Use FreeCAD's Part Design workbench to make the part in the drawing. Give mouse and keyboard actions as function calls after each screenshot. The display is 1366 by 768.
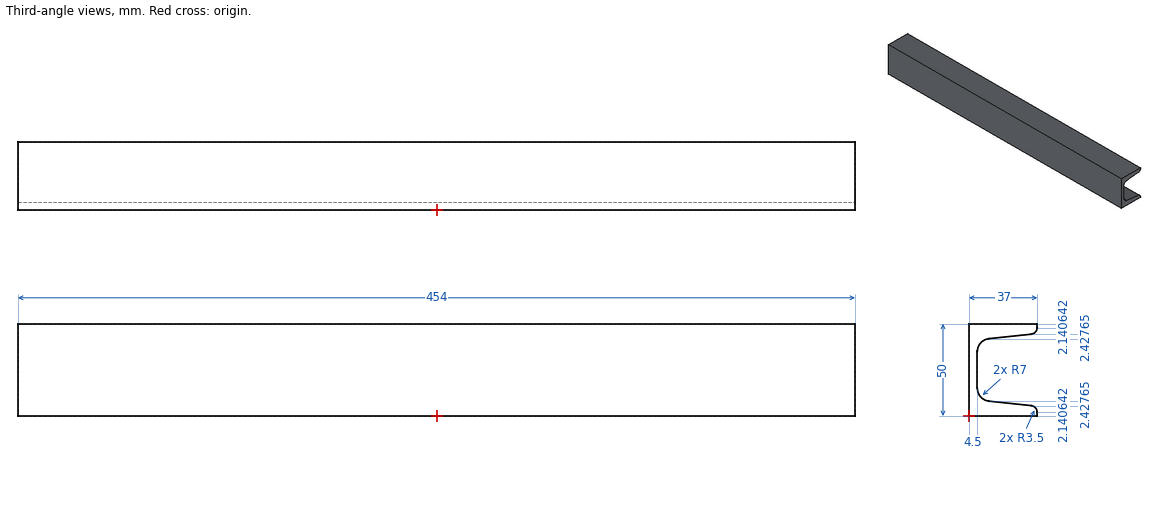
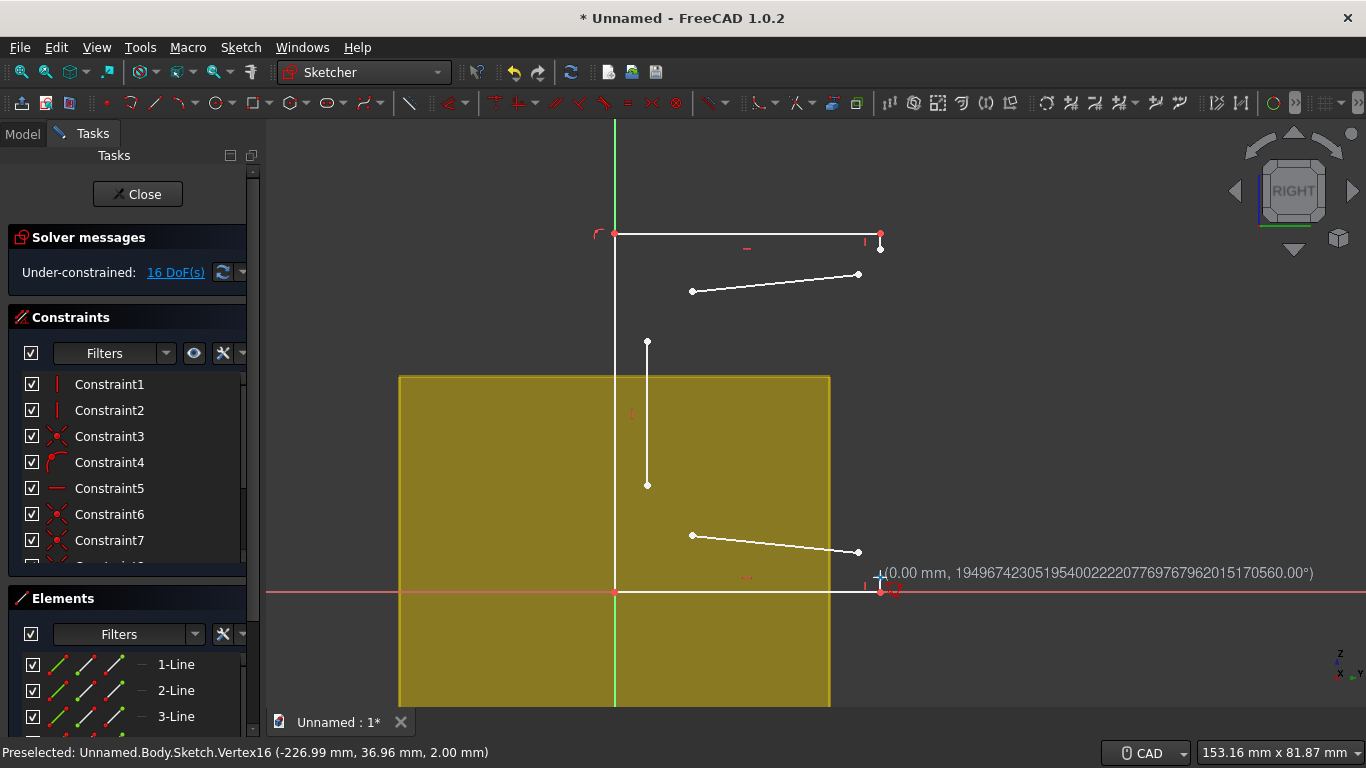
click(180, 104)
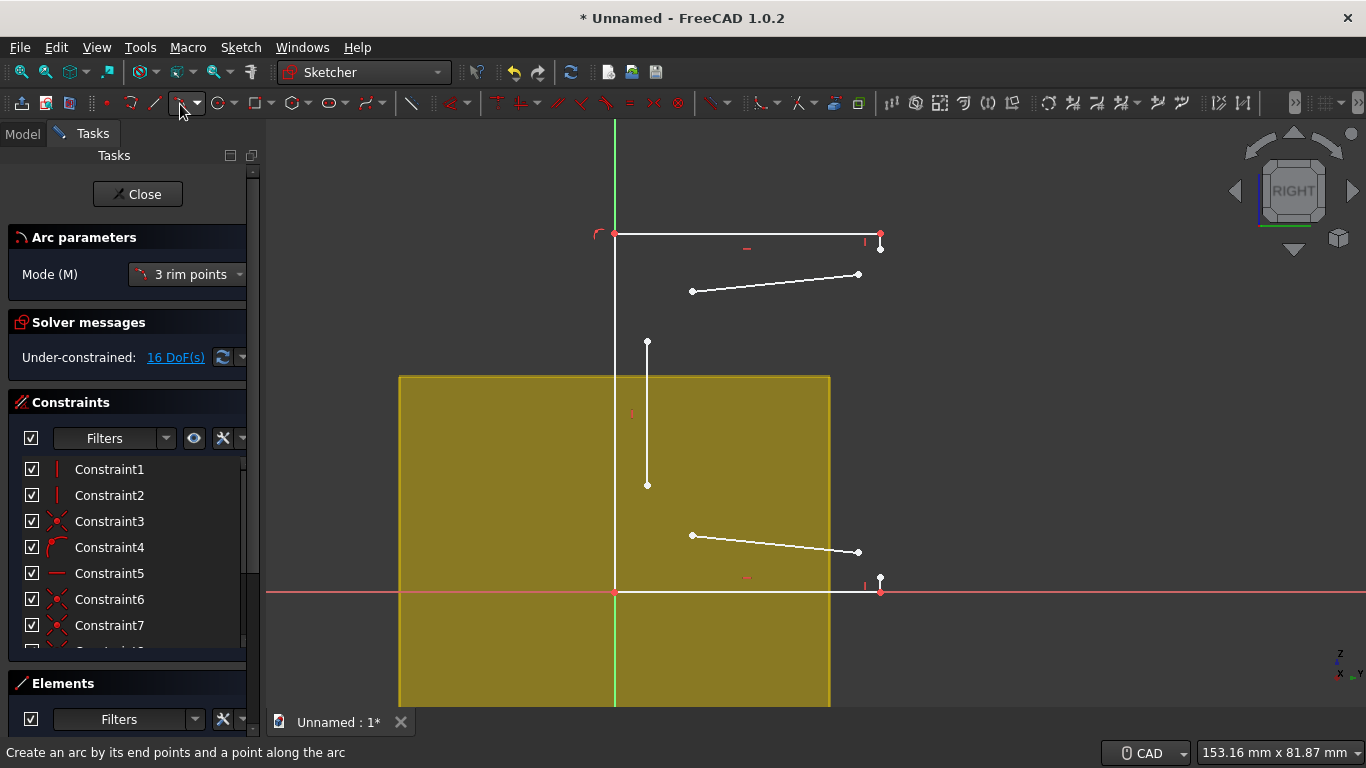
click(692, 536)
click(647, 486)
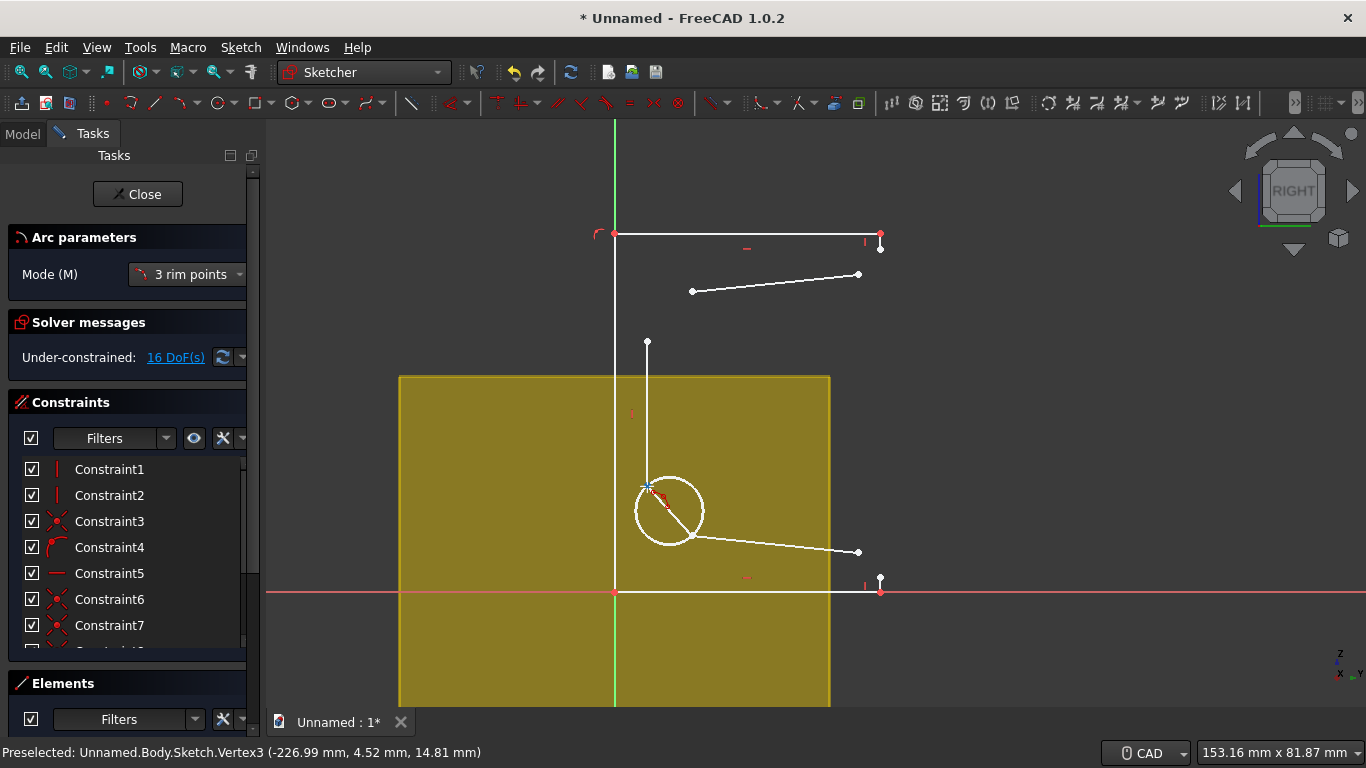
scroll(660, 518, up, 2)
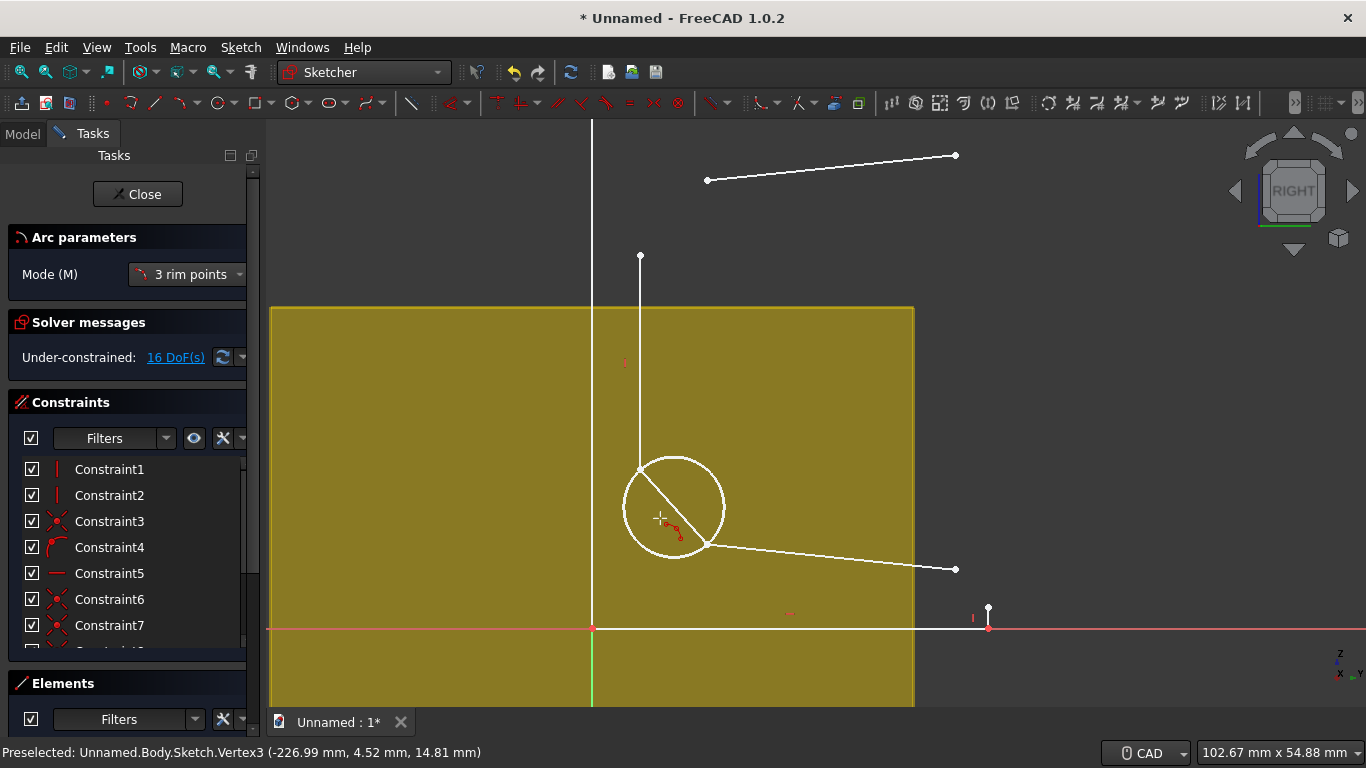
click(659, 518)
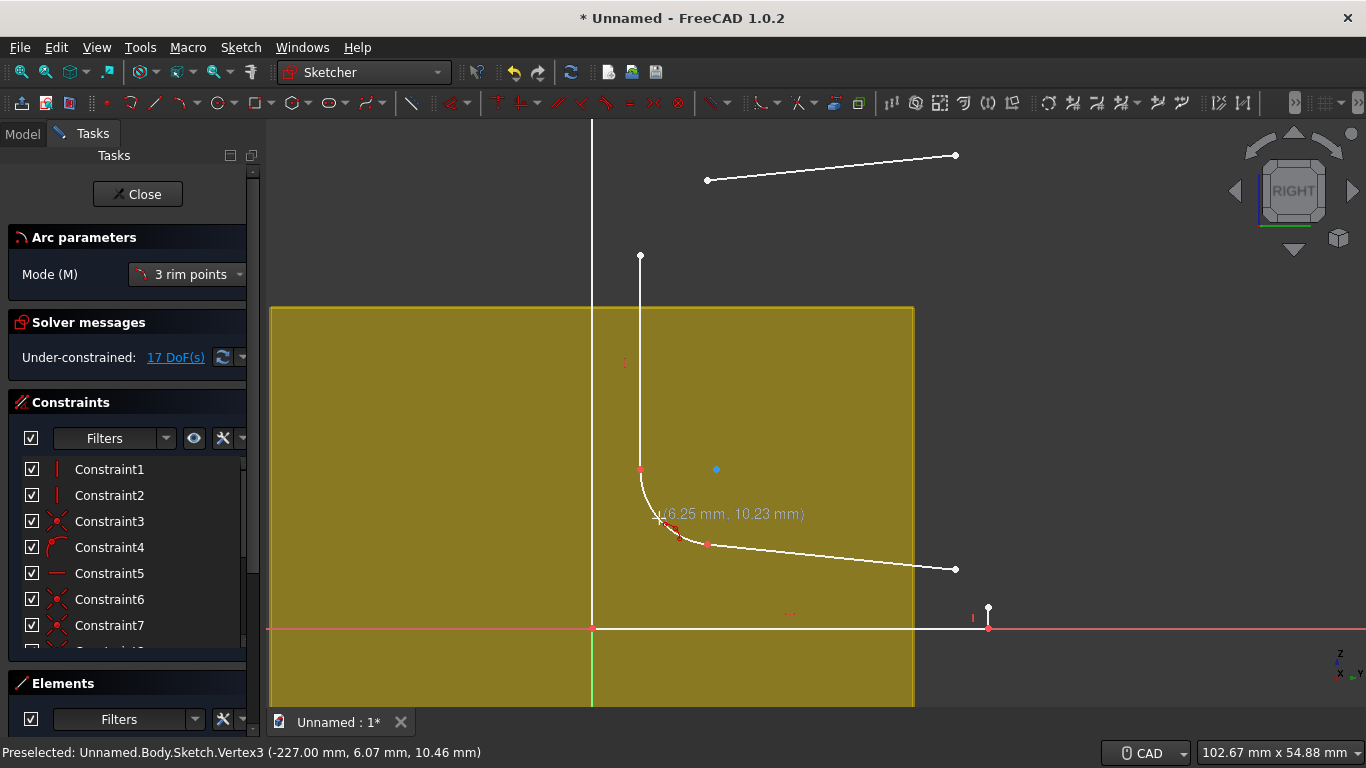
click(640, 255)
click(708, 181)
click(659, 204)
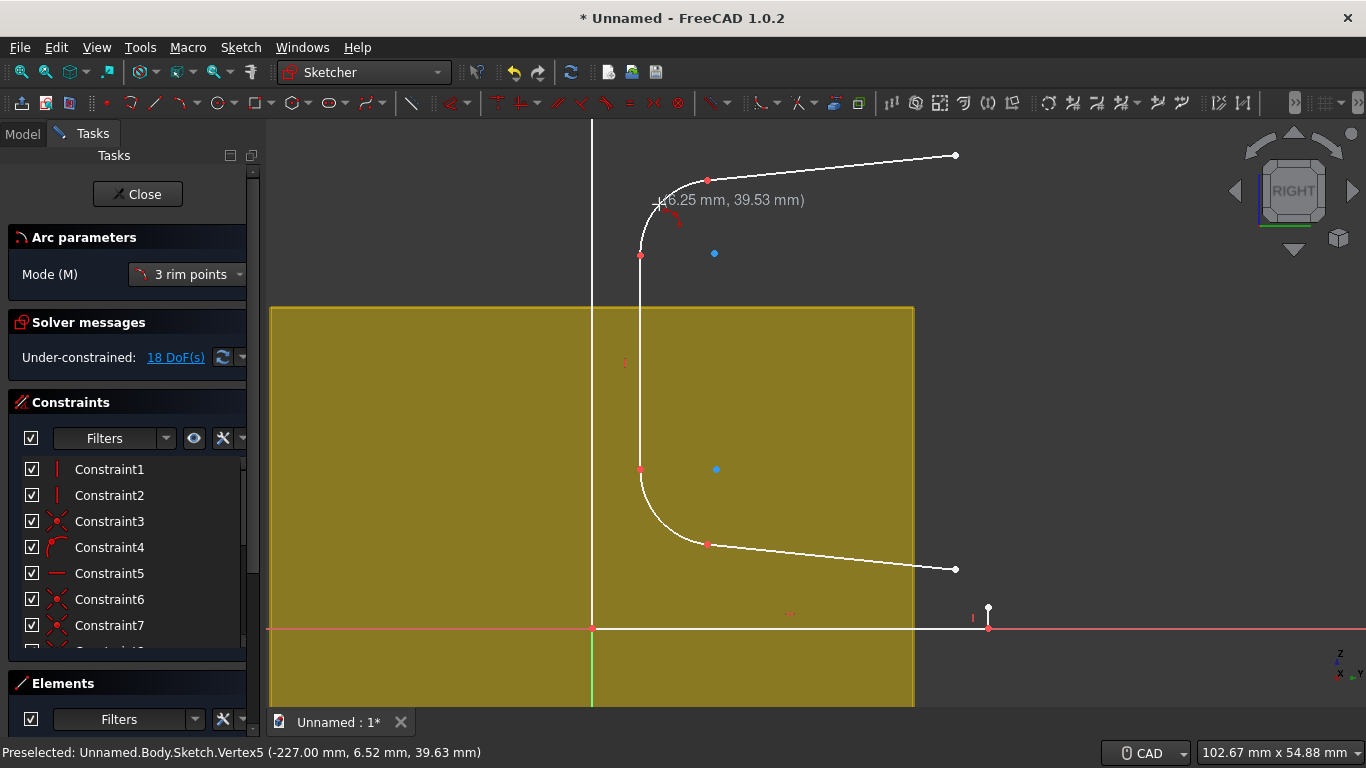
click(955, 155)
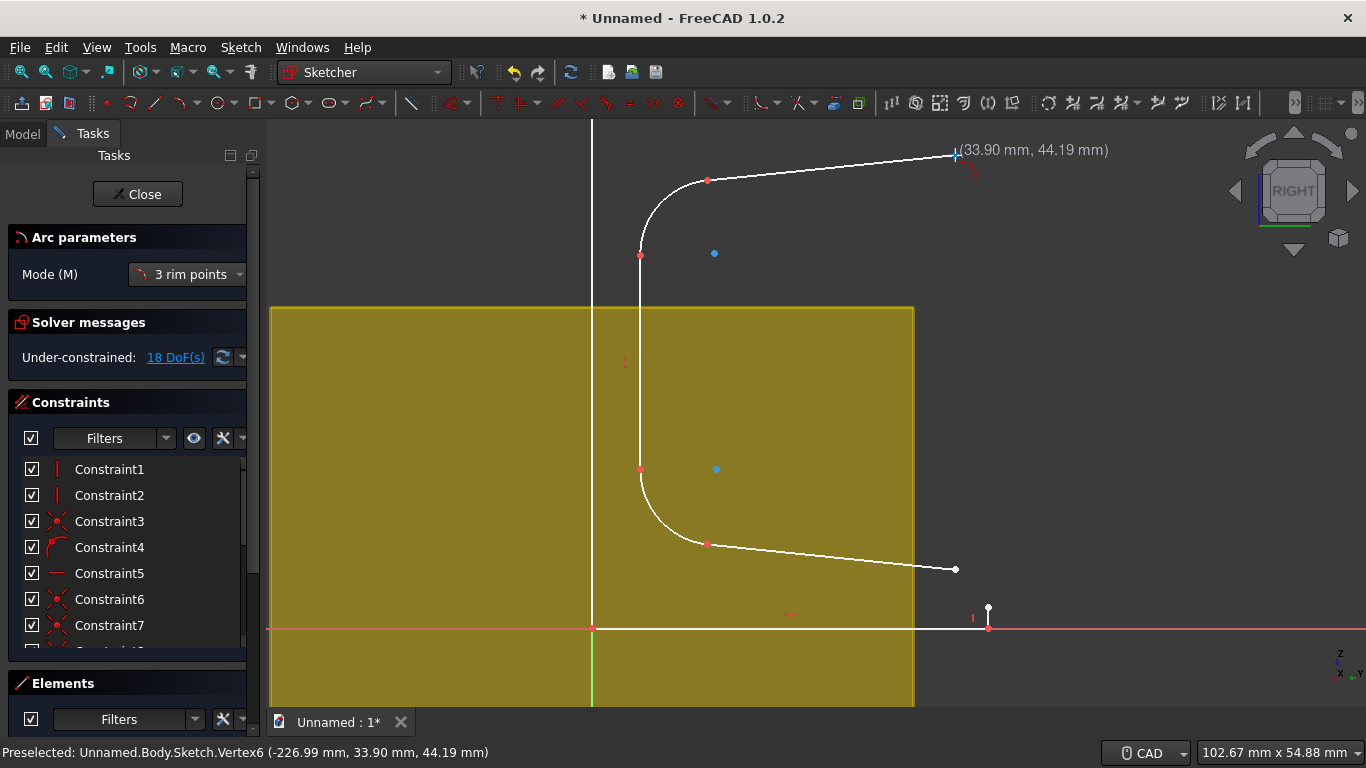
scroll(661, 519, down, 2)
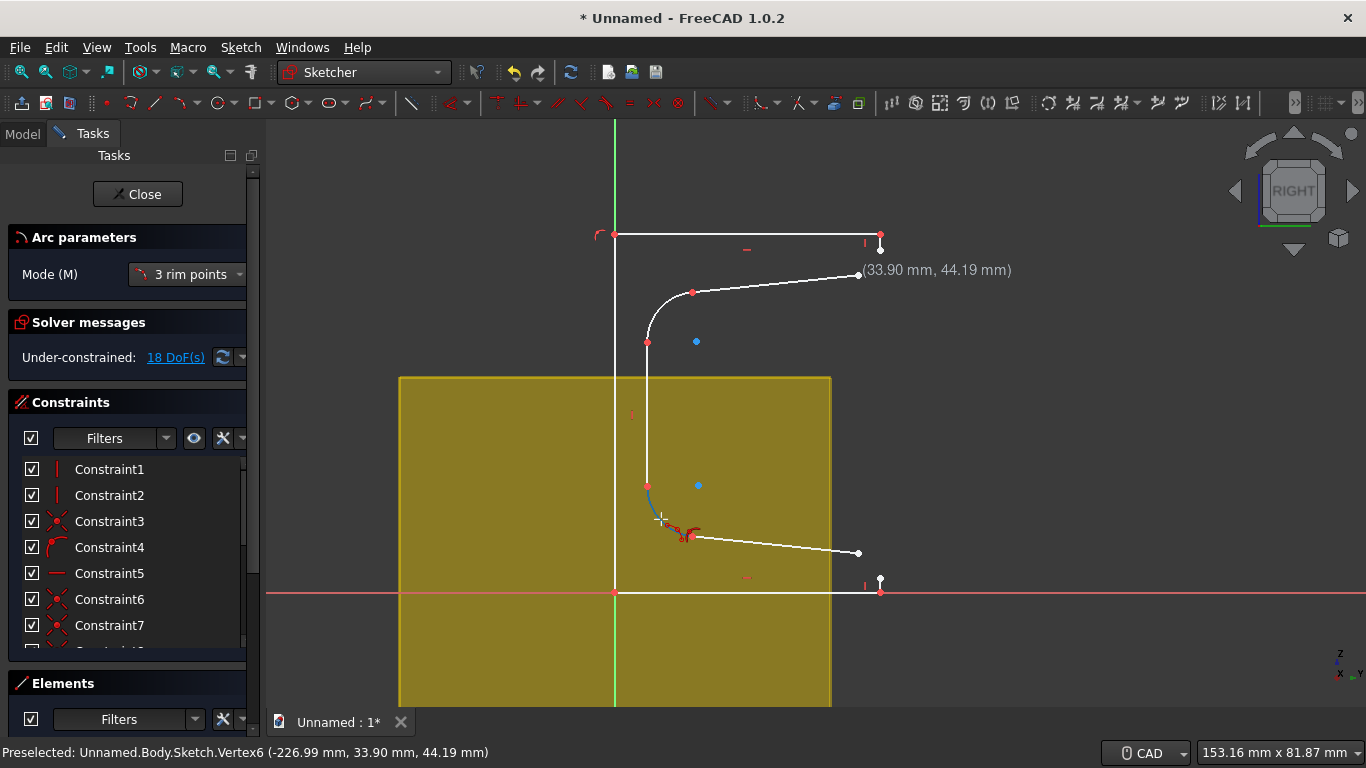
scroll(881, 249, up, 4)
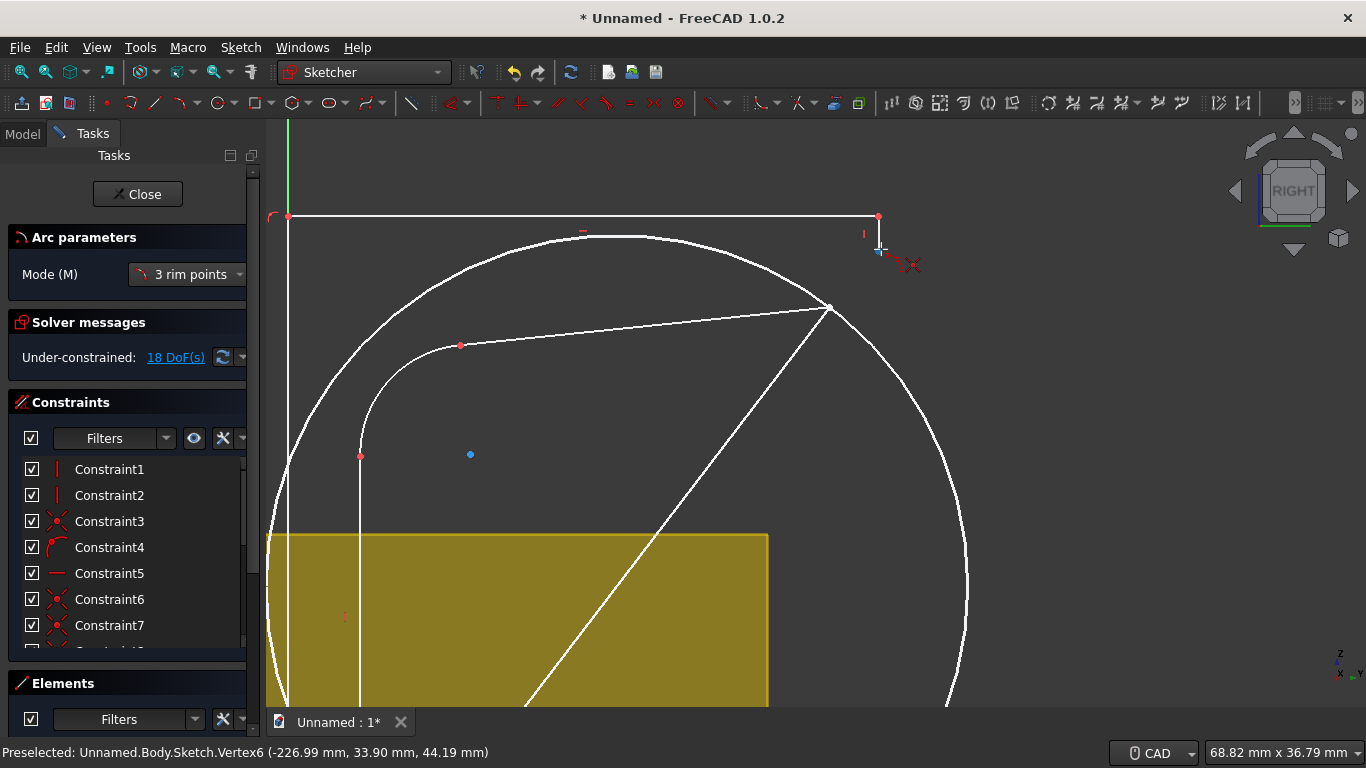
click(879, 252)
click(865, 286)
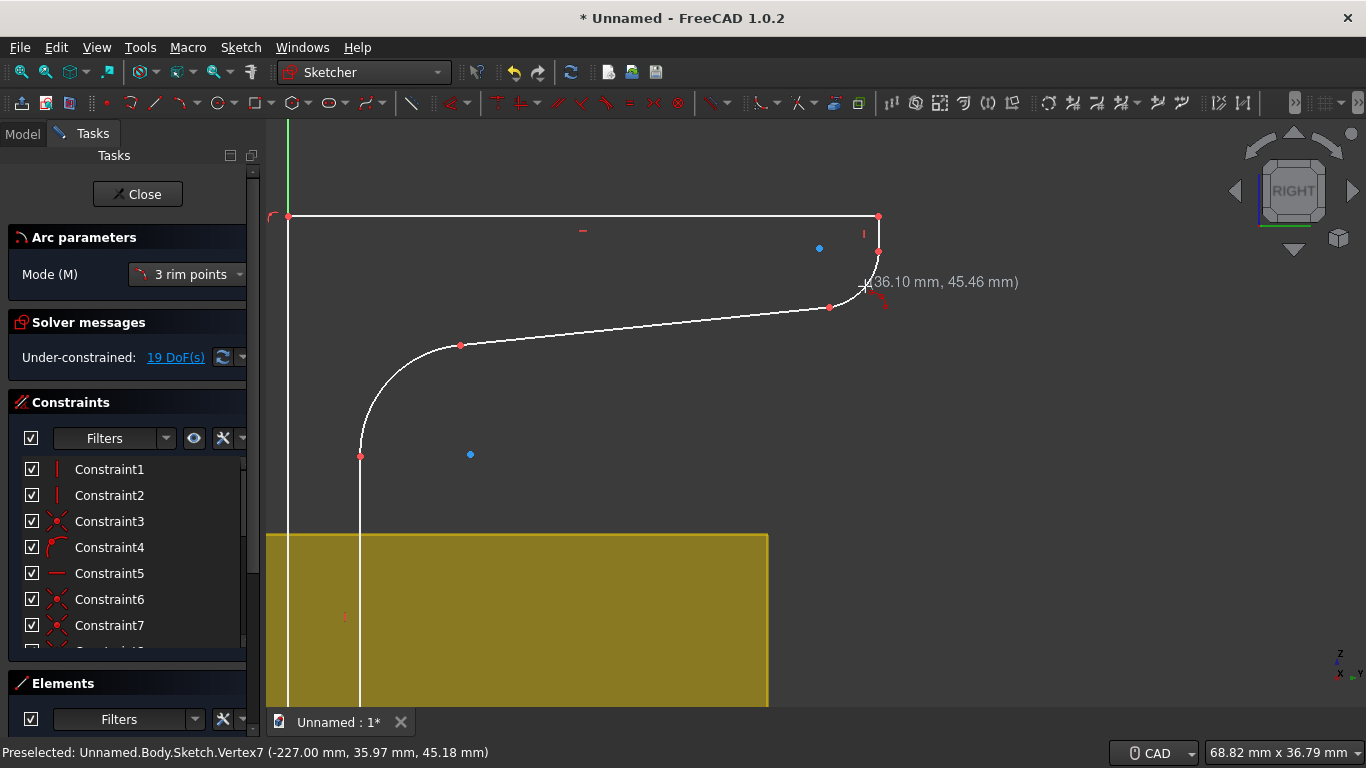
scroll(881, 249, down, 4)